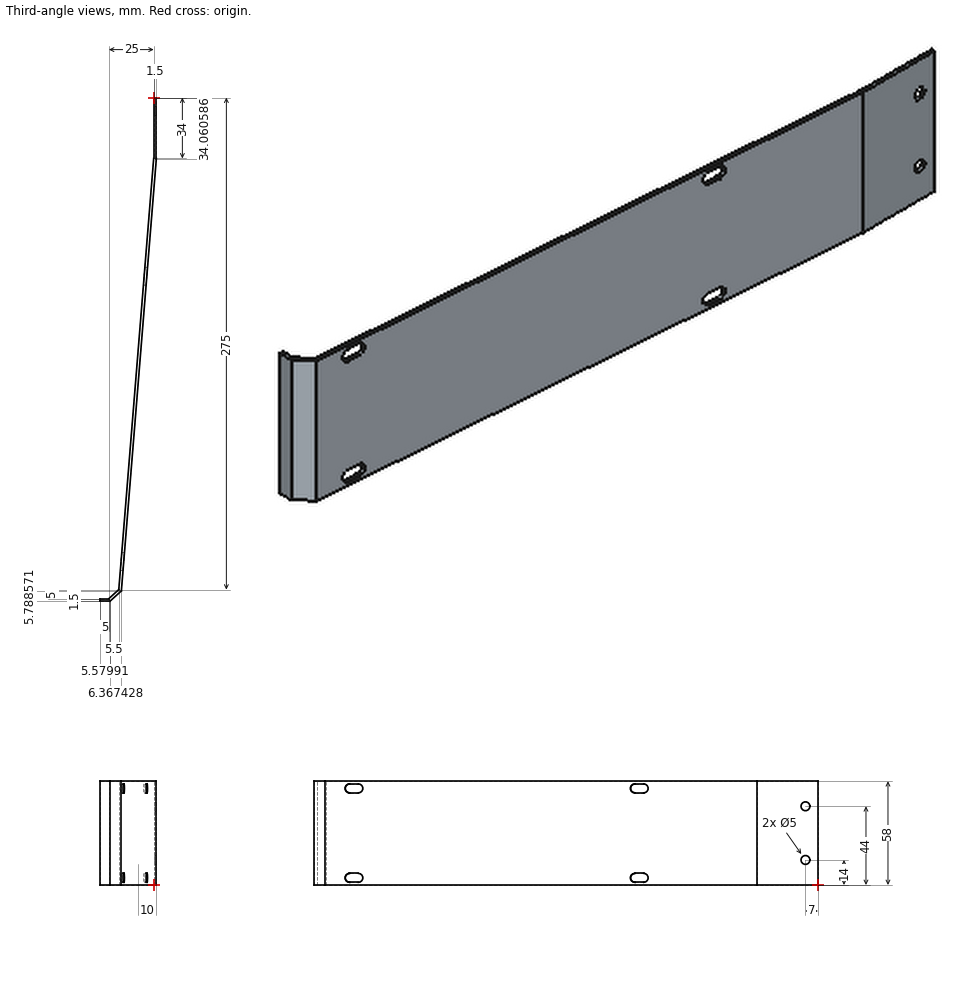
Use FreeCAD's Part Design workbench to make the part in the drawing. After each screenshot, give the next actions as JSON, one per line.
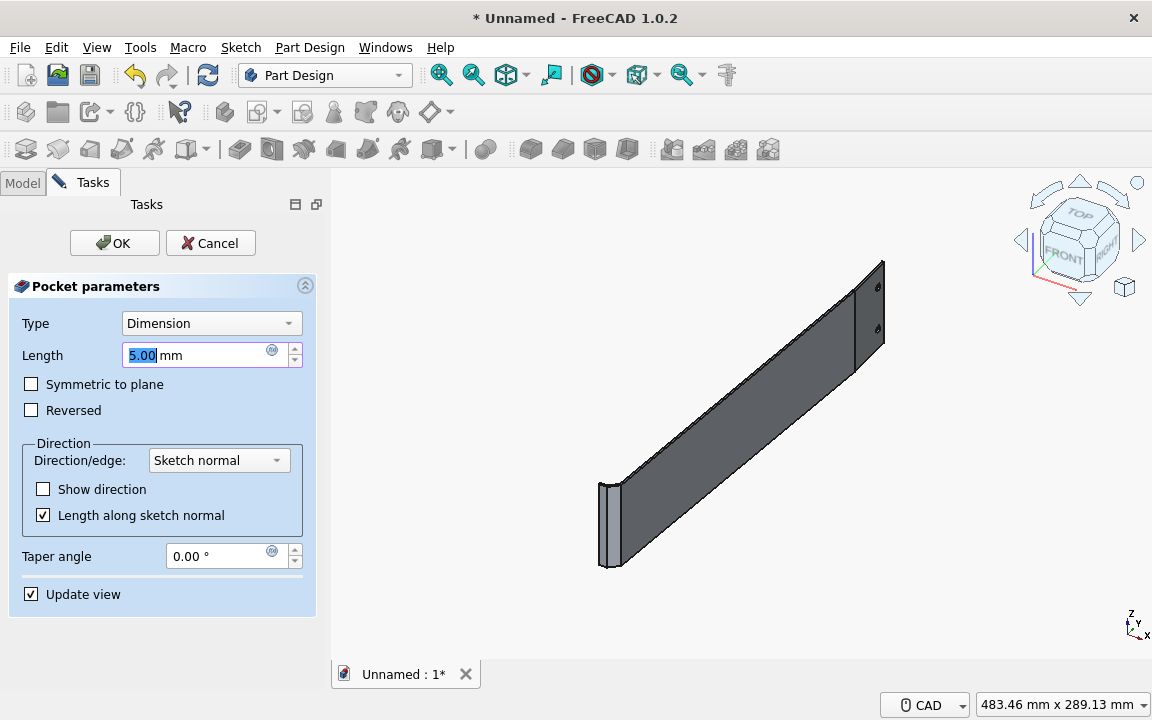
{"action": "type", "text": "10"}
{"action": "key", "text": "Tab"}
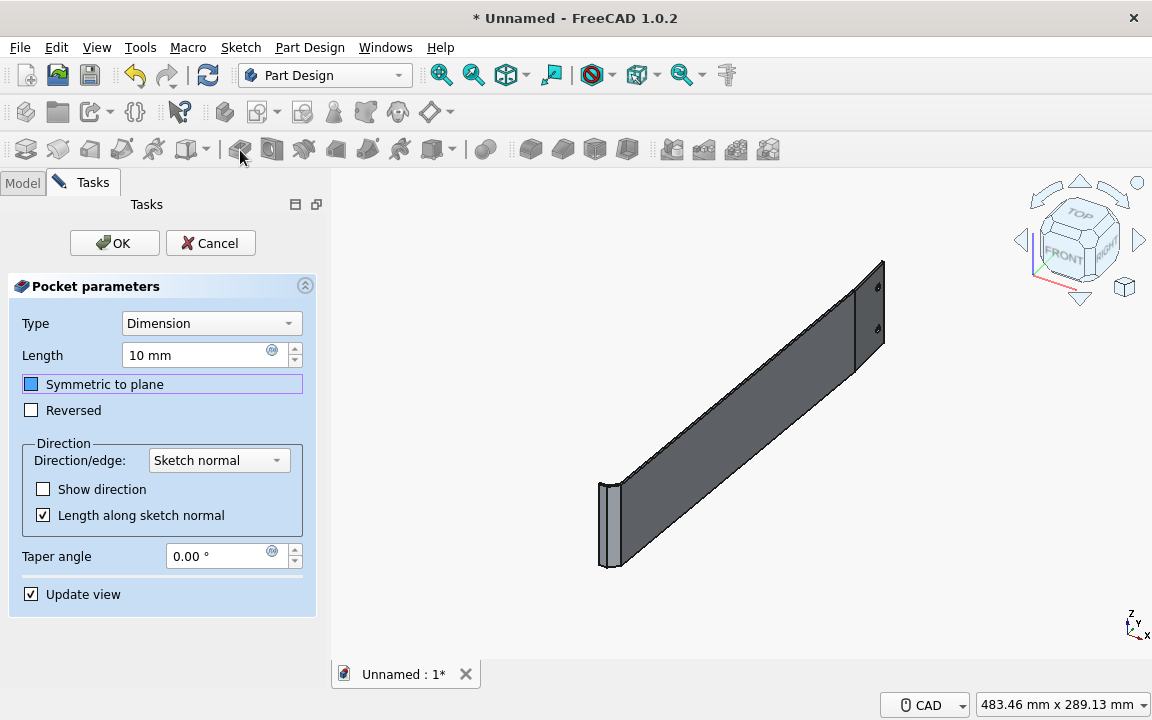
{"action": "left_click", "coordinate": [115, 243]}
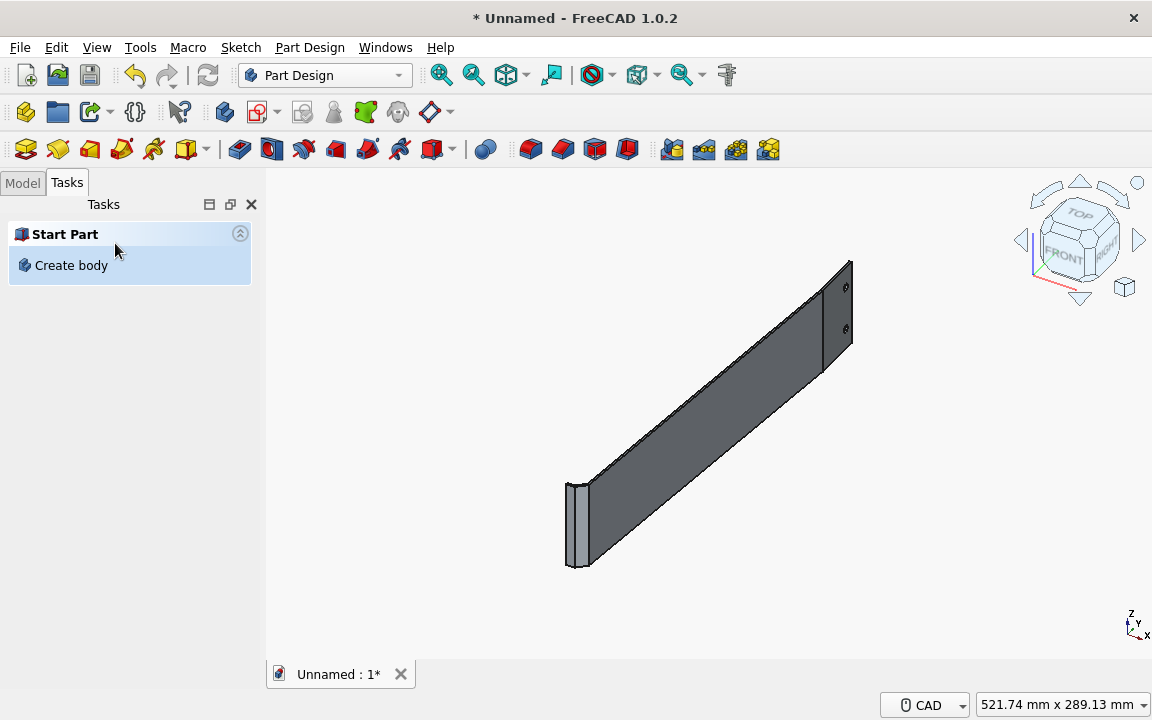
{"action": "left_click", "coordinate": [773, 372]}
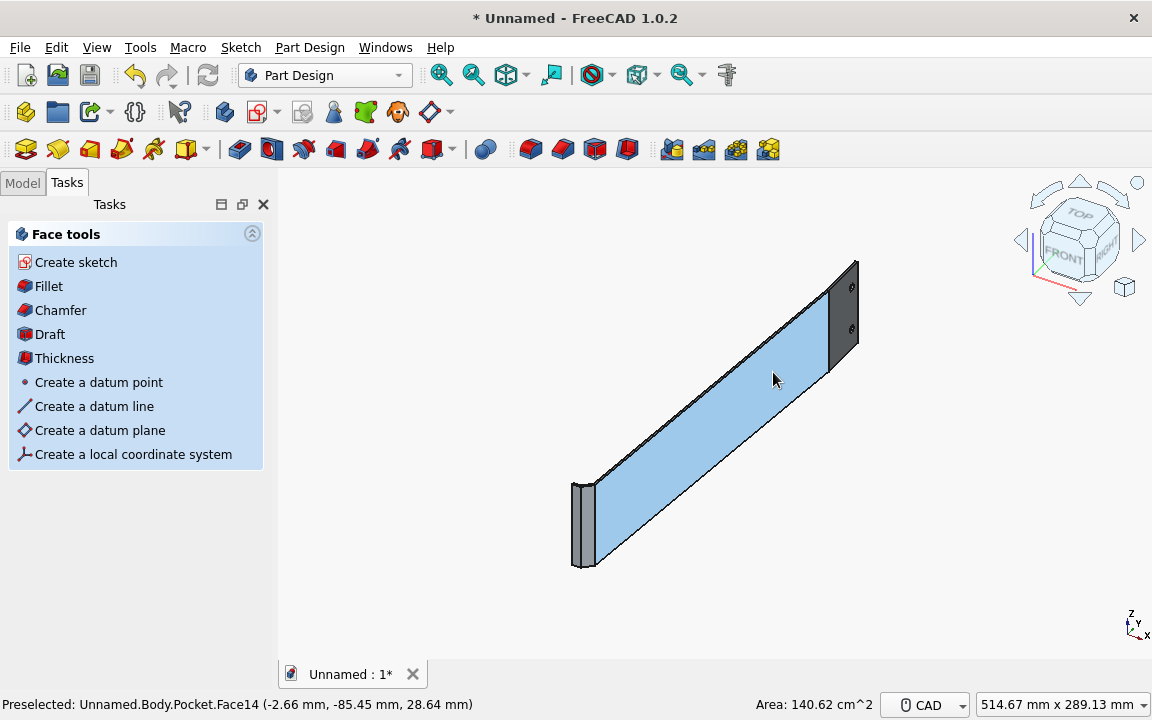
{"action": "left_click", "coordinate": [258, 112]}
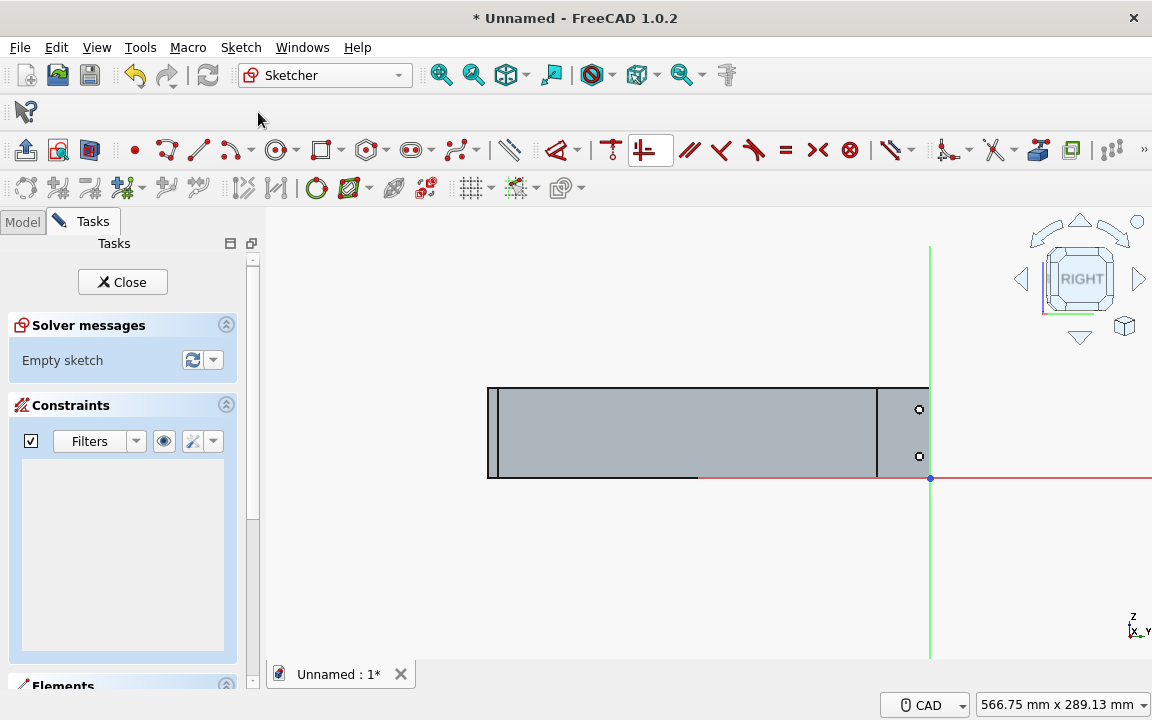
{"action": "left_click", "coordinate": [412, 150]}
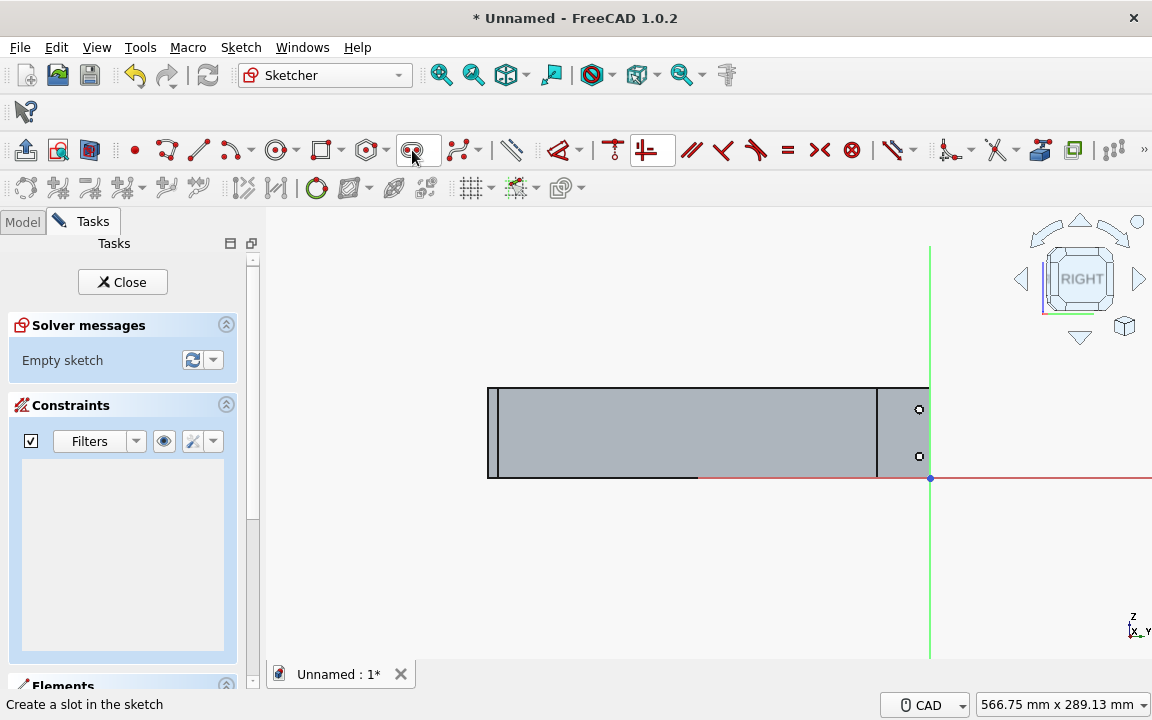
{"action": "scroll", "coordinate": [770, 394], "scroll_direction": "up", "scroll_amount": 9}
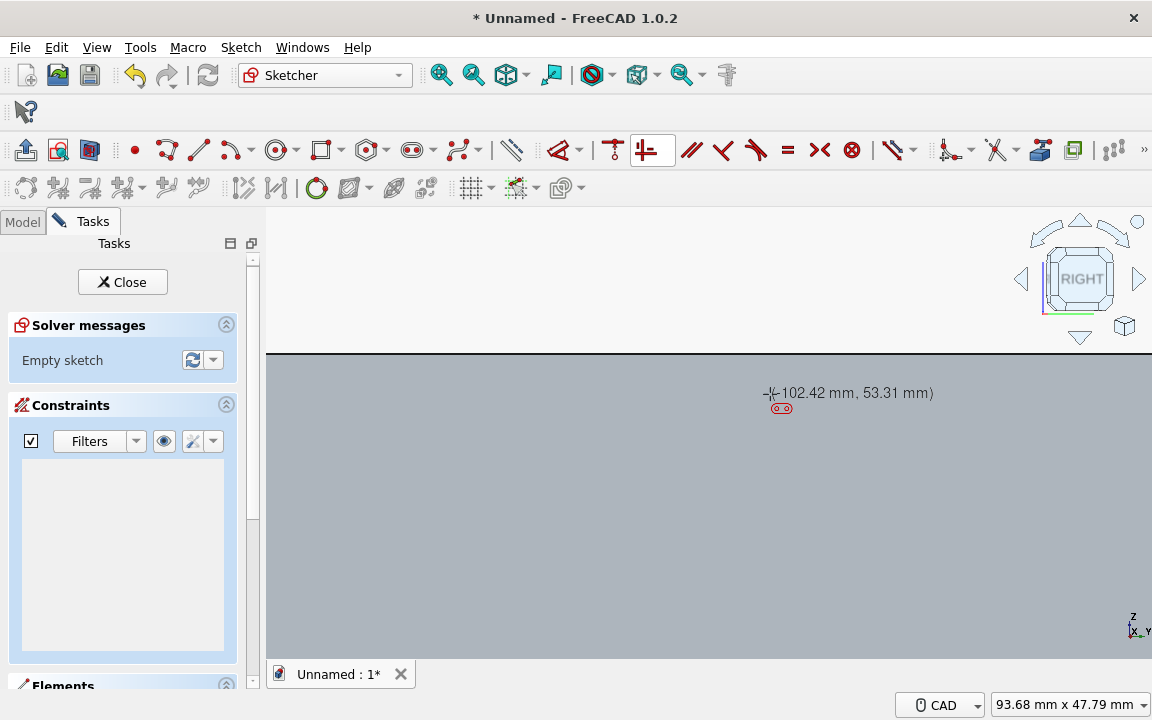
{"action": "scroll", "coordinate": [680, 382], "scroll_direction": "down", "scroll_amount": 8}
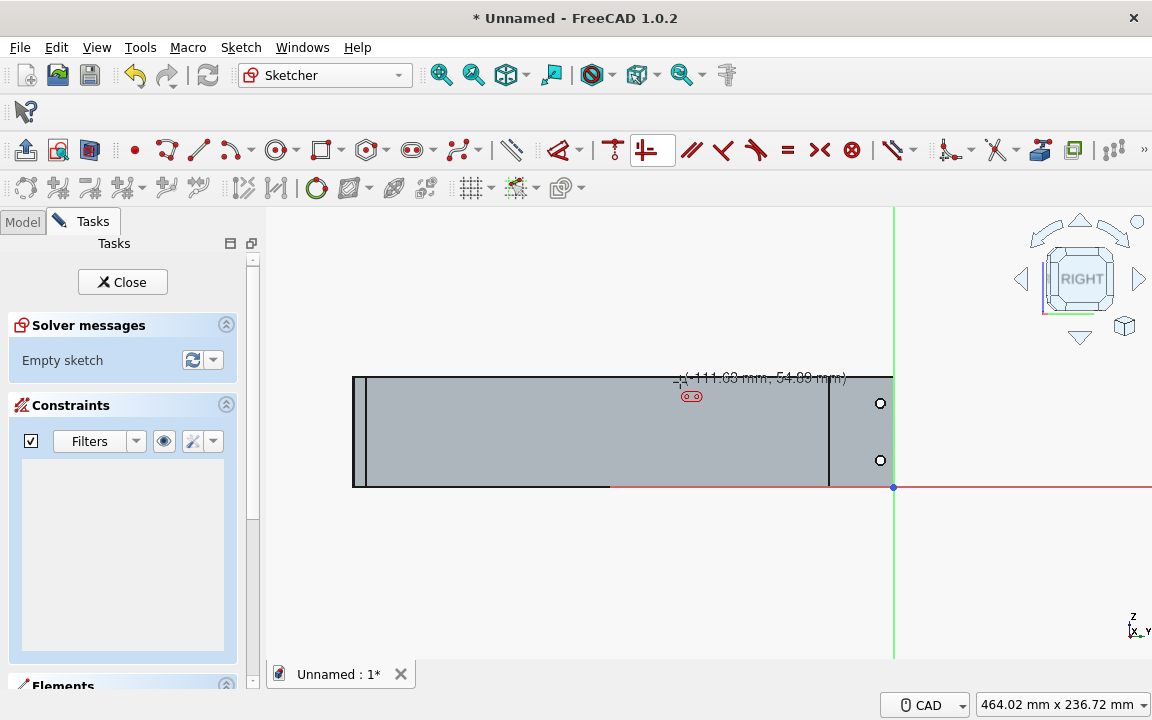
{"action": "left_click", "coordinate": [698, 384]}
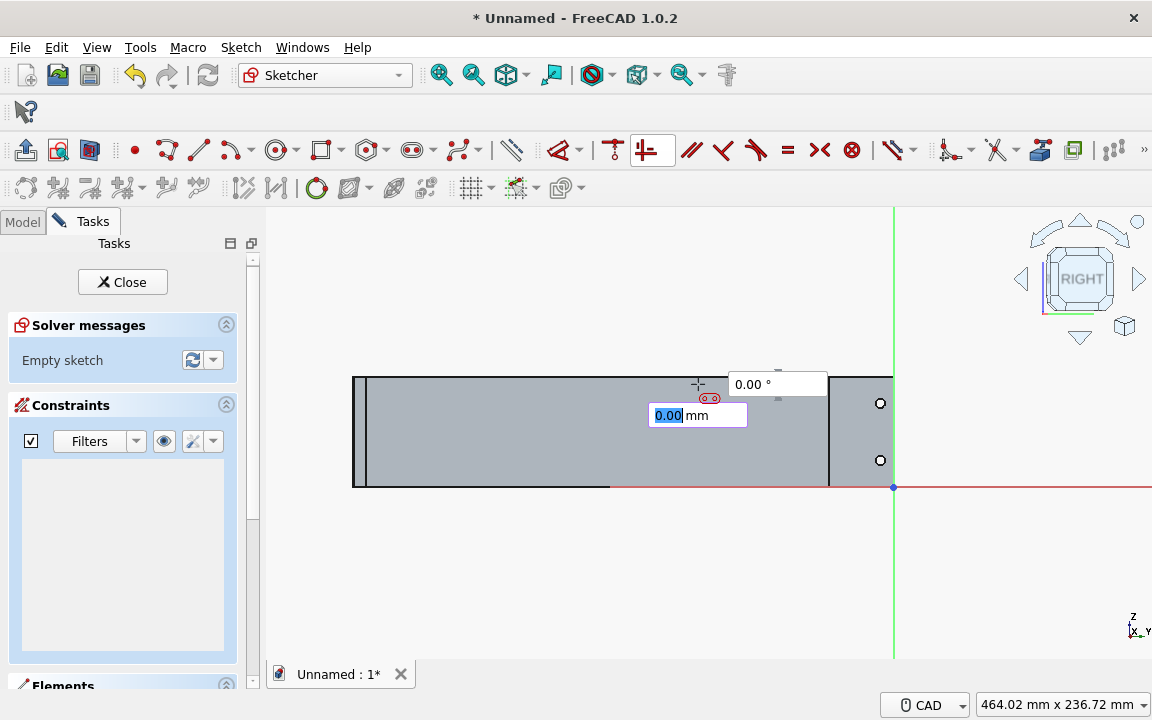
{"action": "scroll", "coordinate": [708, 384], "scroll_direction": "up", "scroll_amount": 3}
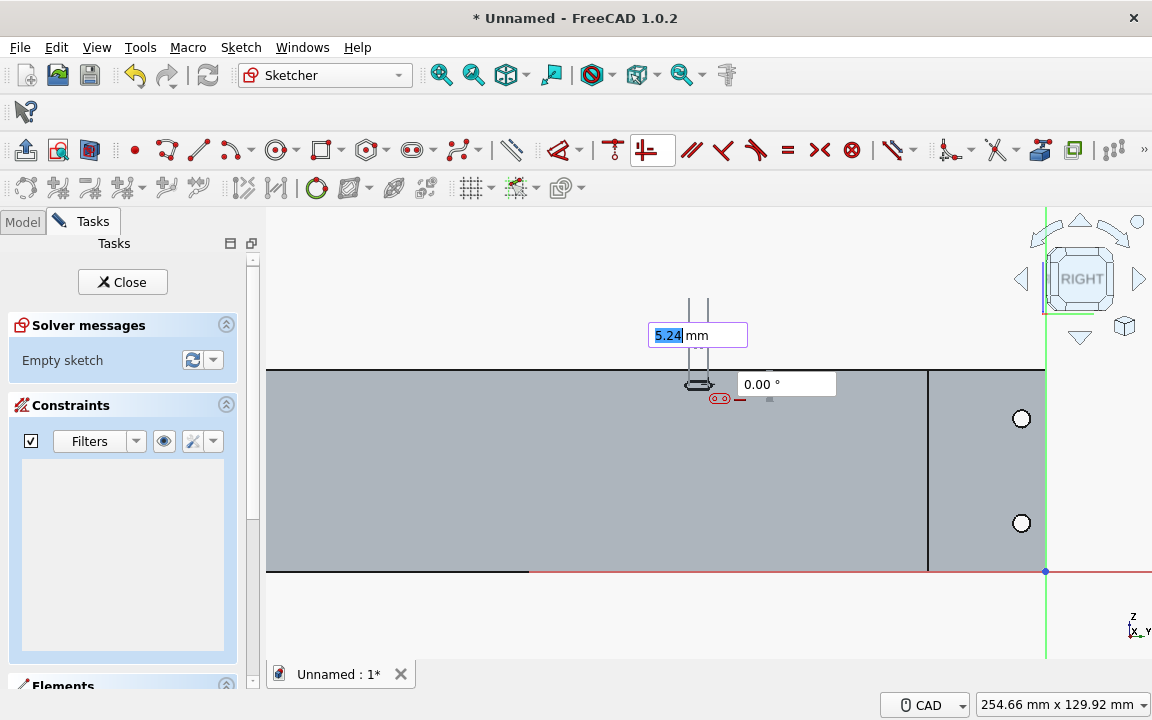
{"action": "left_click", "coordinate": [707, 384]}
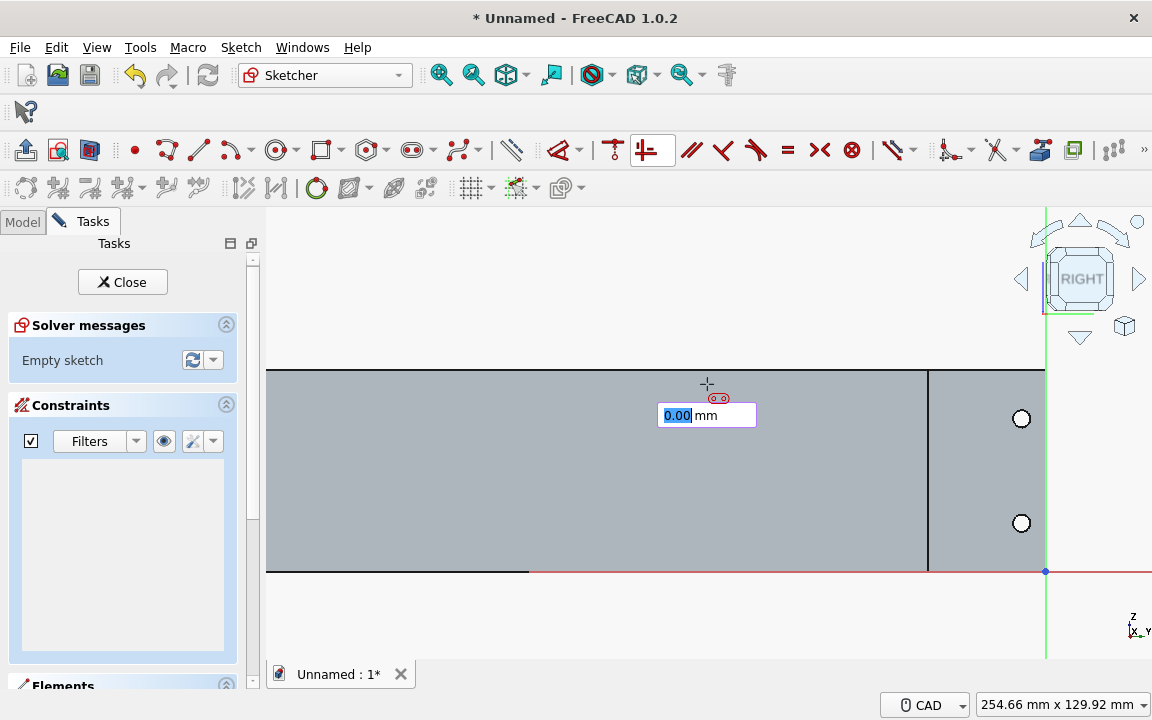
{"action": "scroll", "coordinate": [698, 393], "scroll_direction": "up", "scroll_amount": 4}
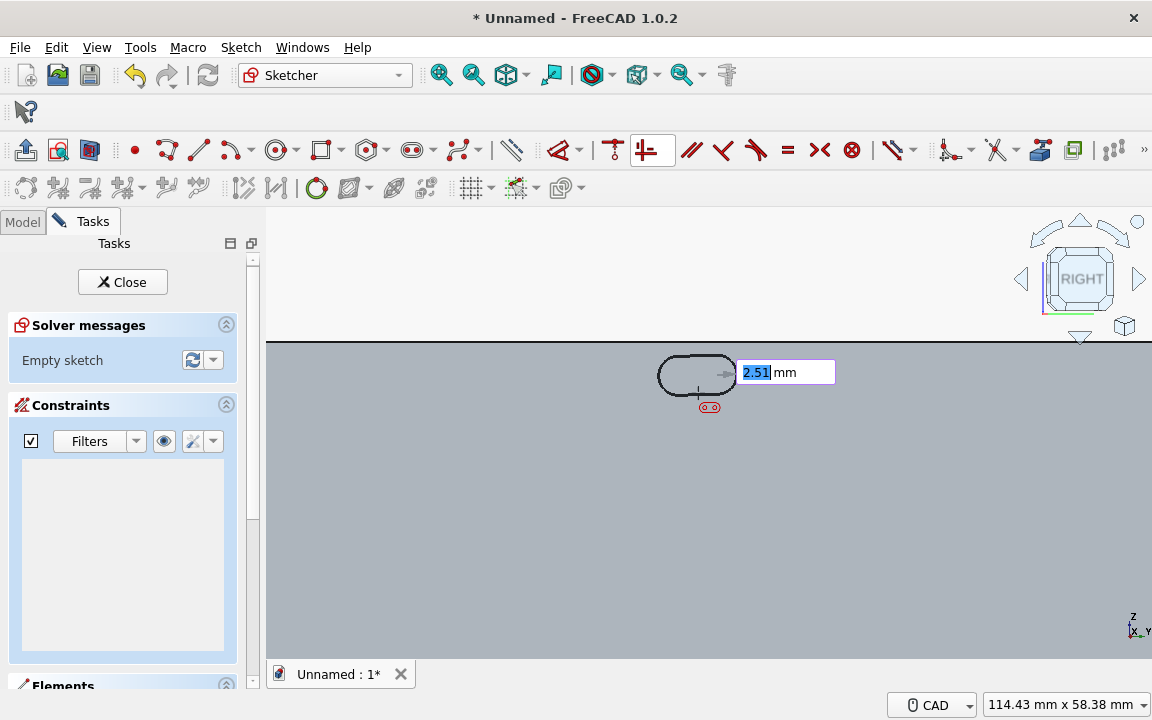
{"action": "left_click", "coordinate": [698, 392]}